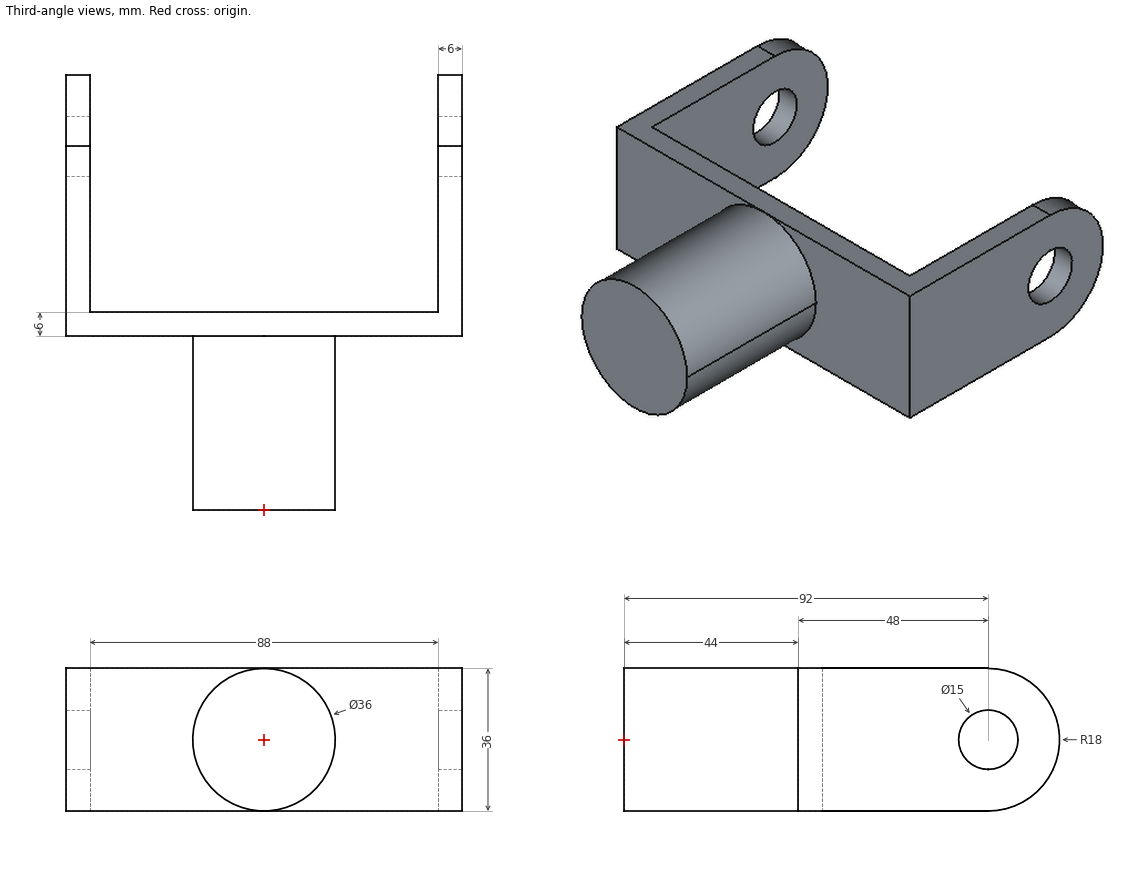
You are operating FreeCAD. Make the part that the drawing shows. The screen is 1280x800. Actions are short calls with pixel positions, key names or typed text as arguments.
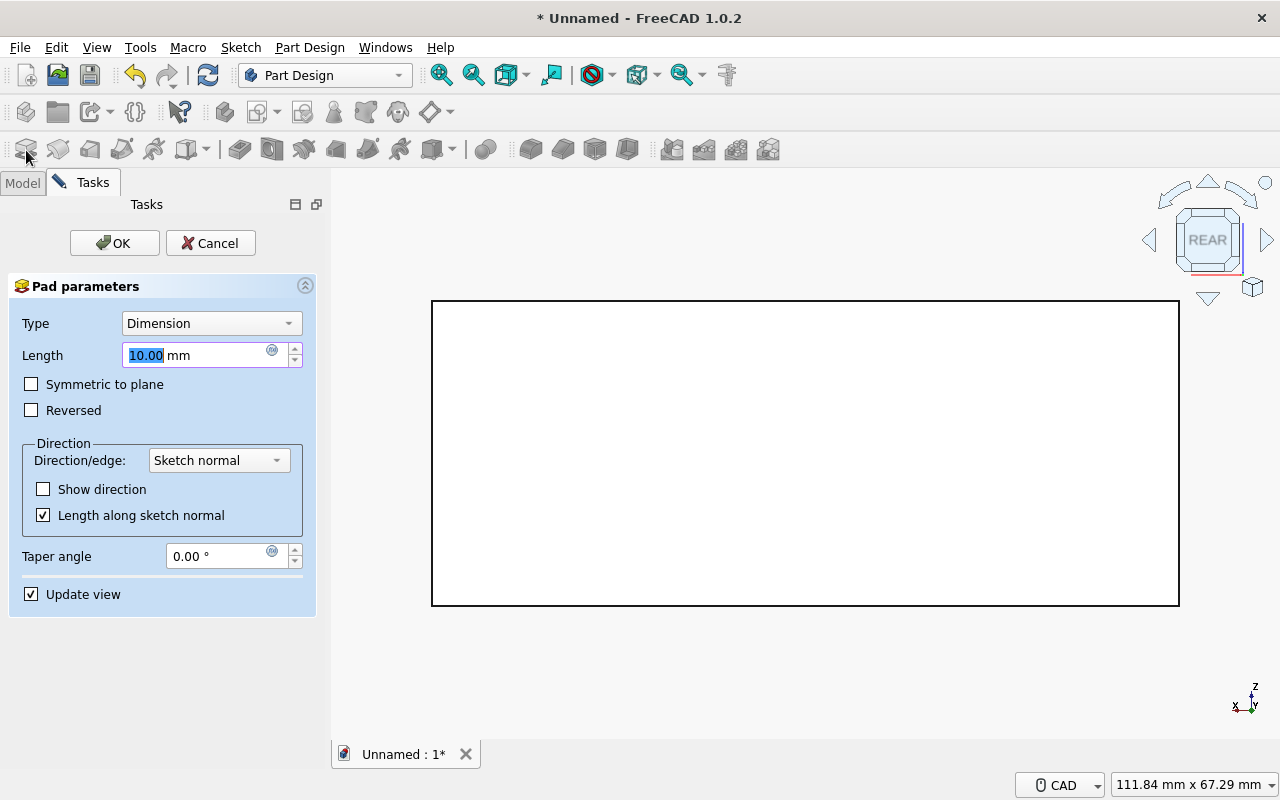
text(6)
key(Tab)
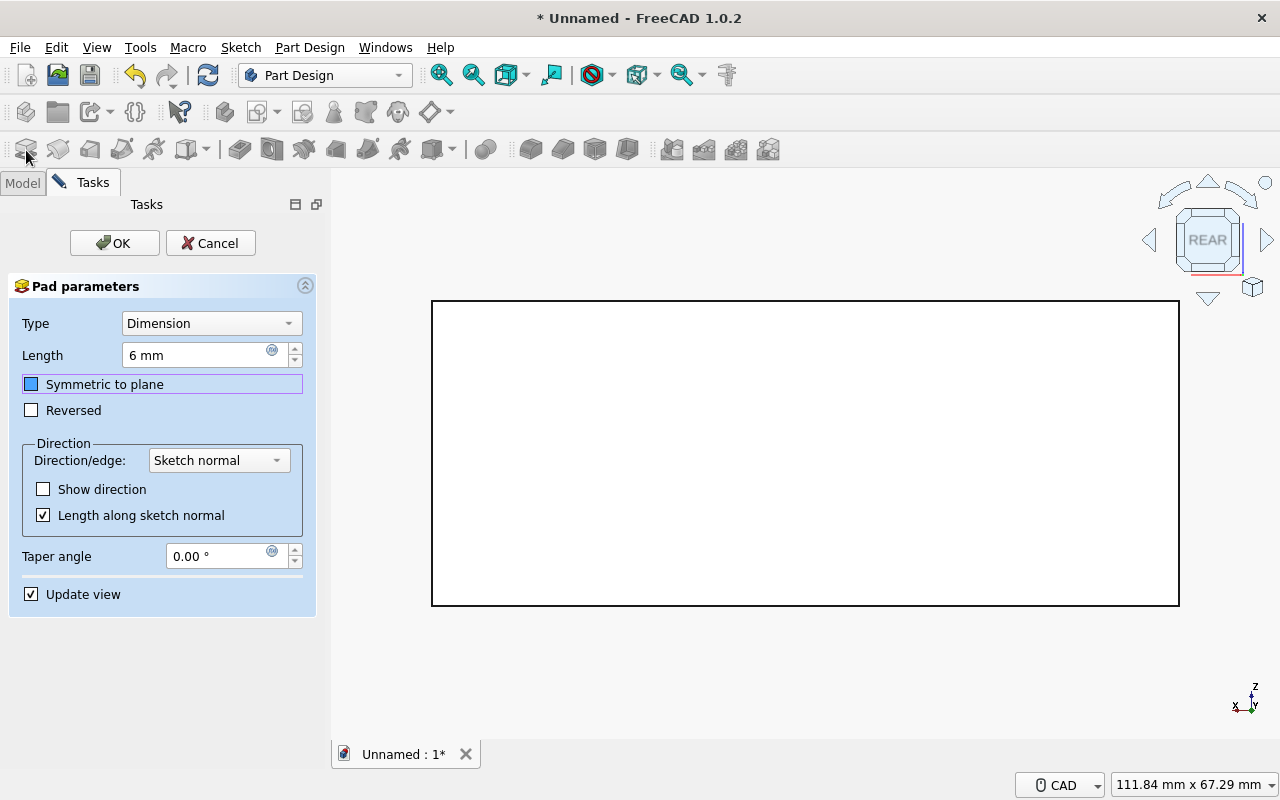
click(115, 243)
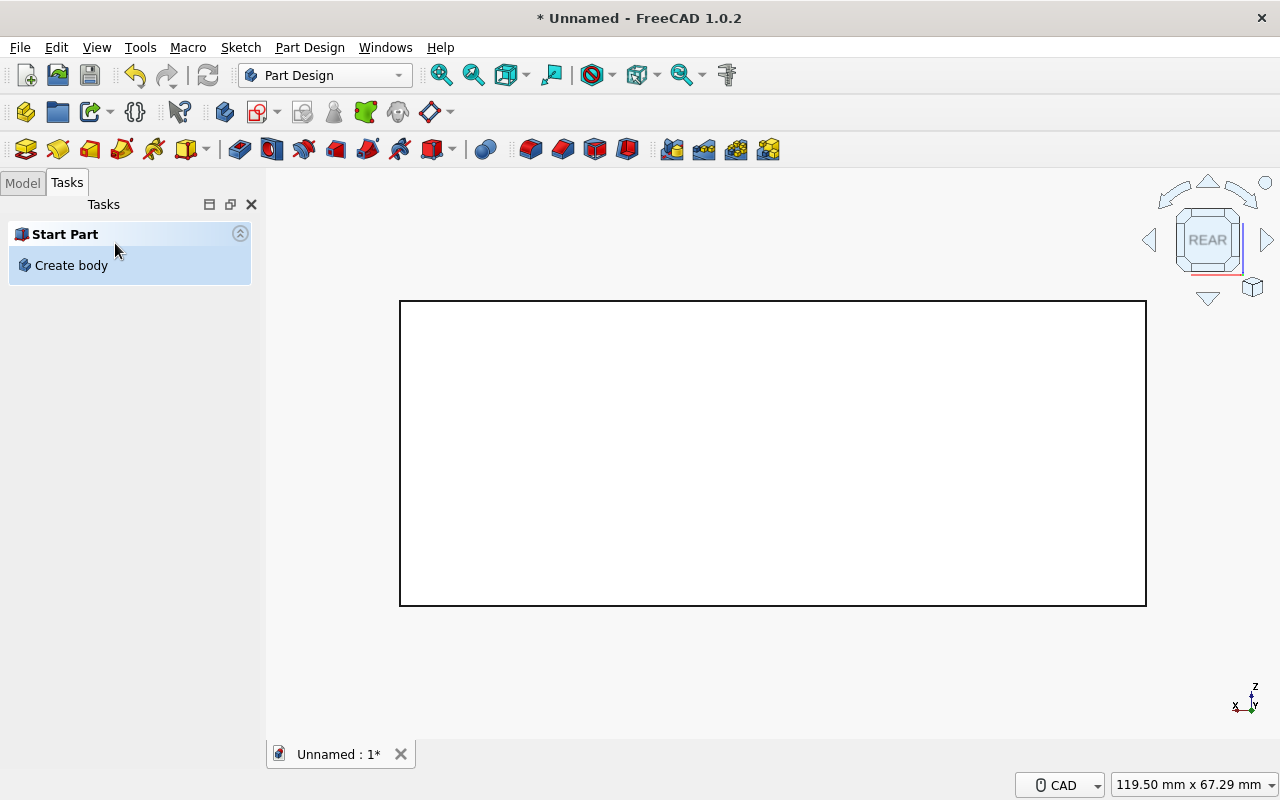
key(0)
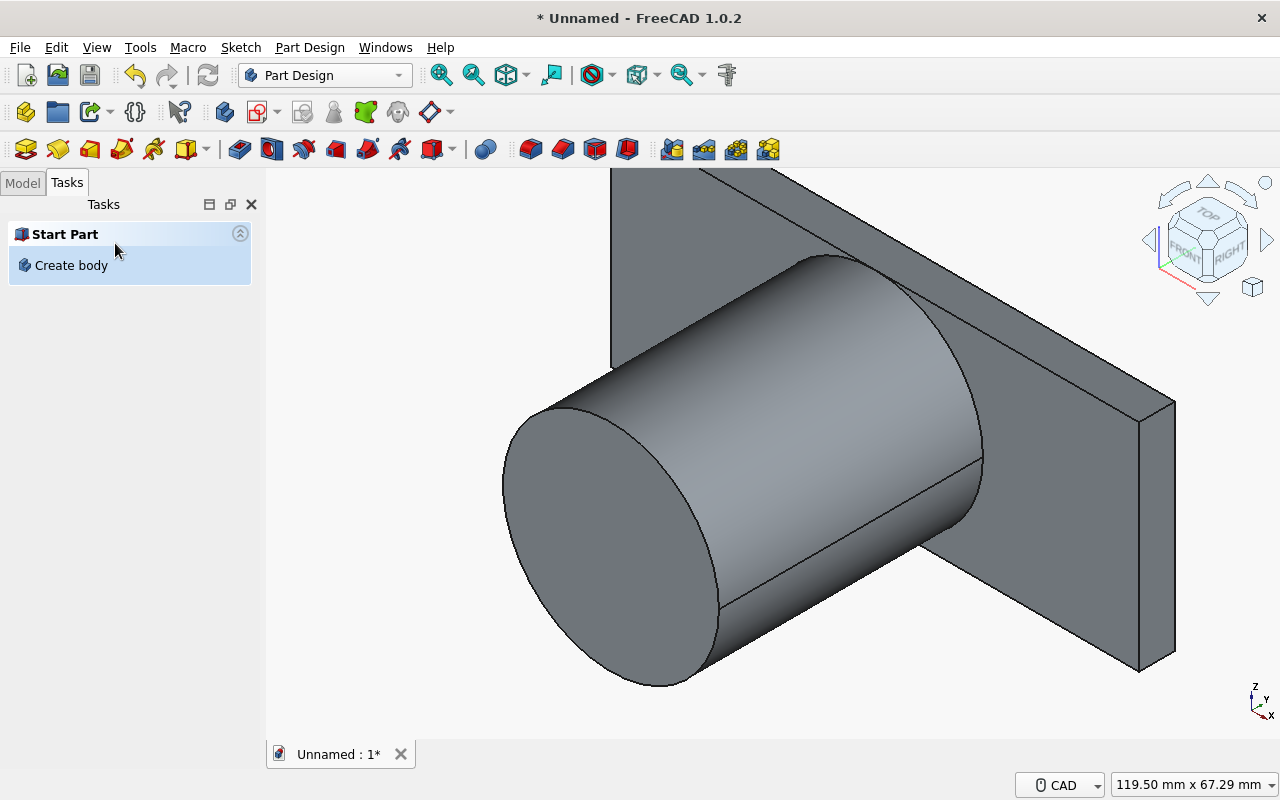
key(v)
key(f)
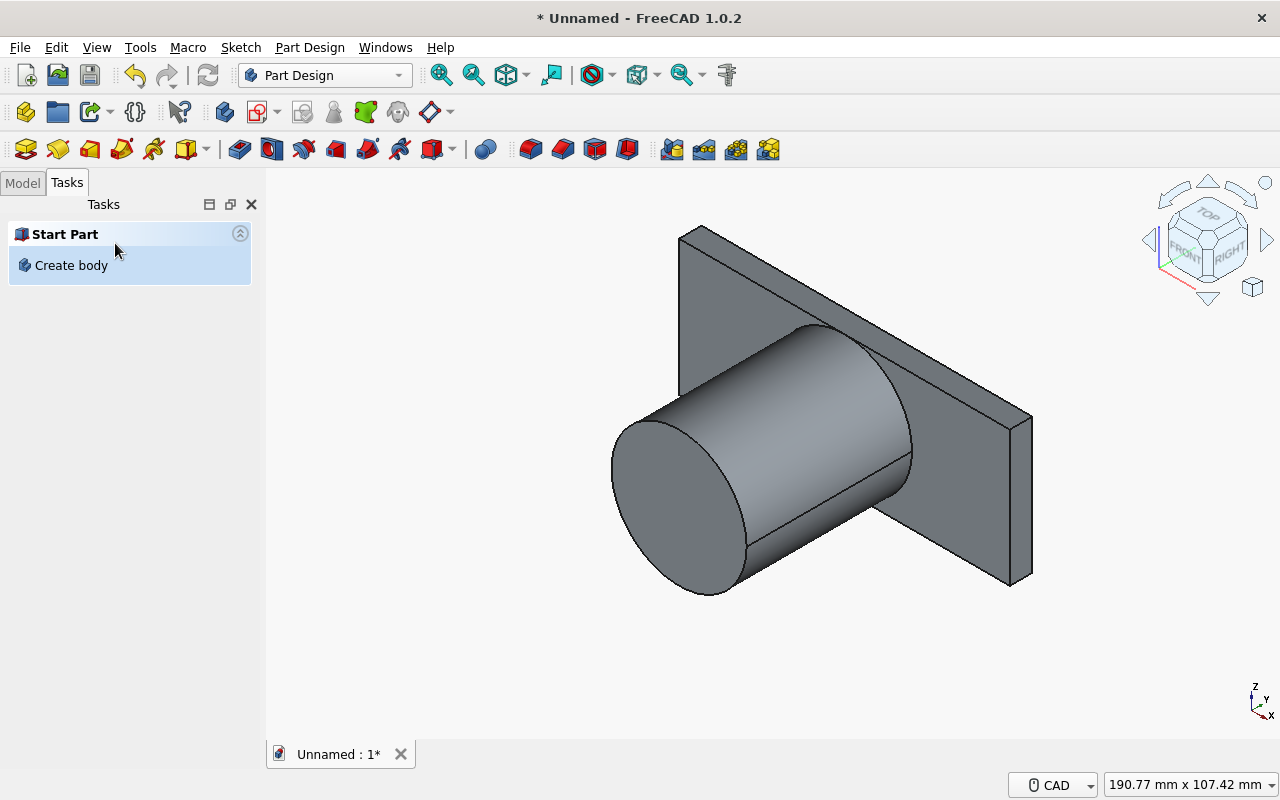
click(1021, 500)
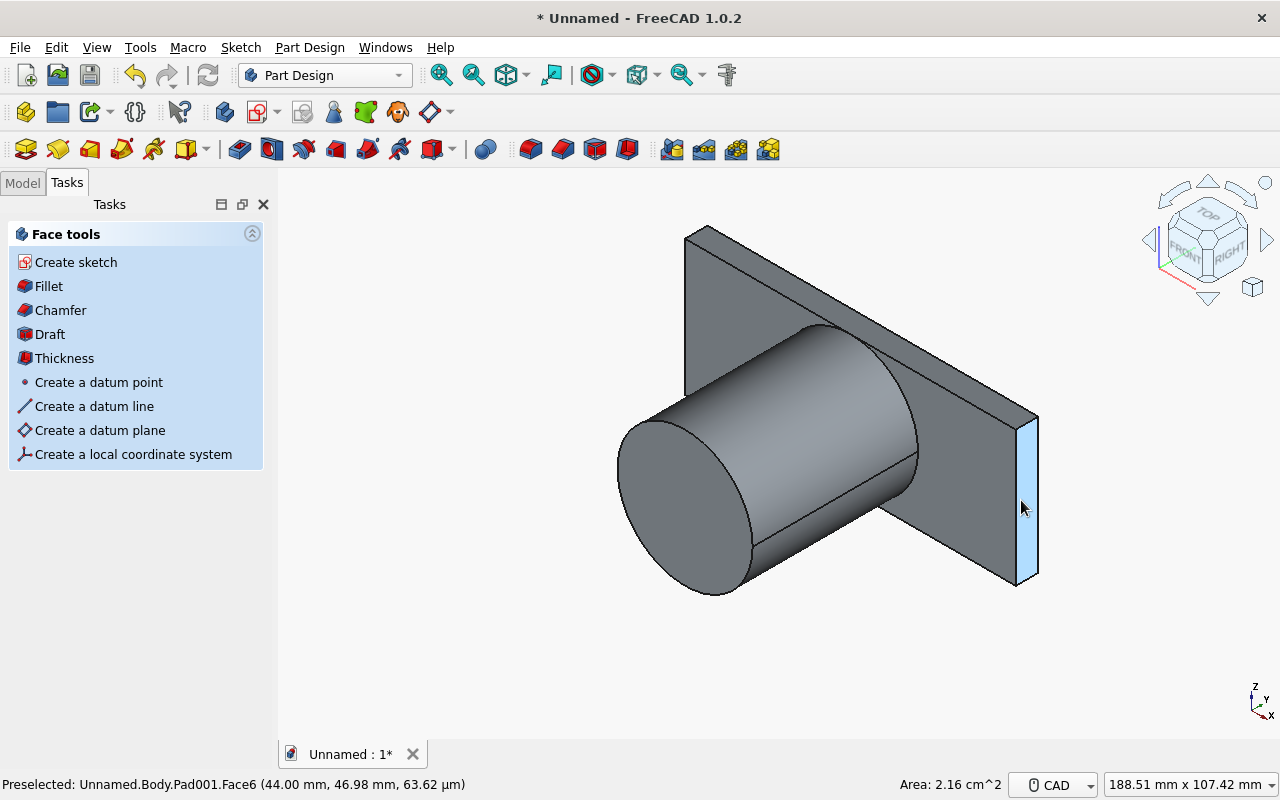
click(258, 112)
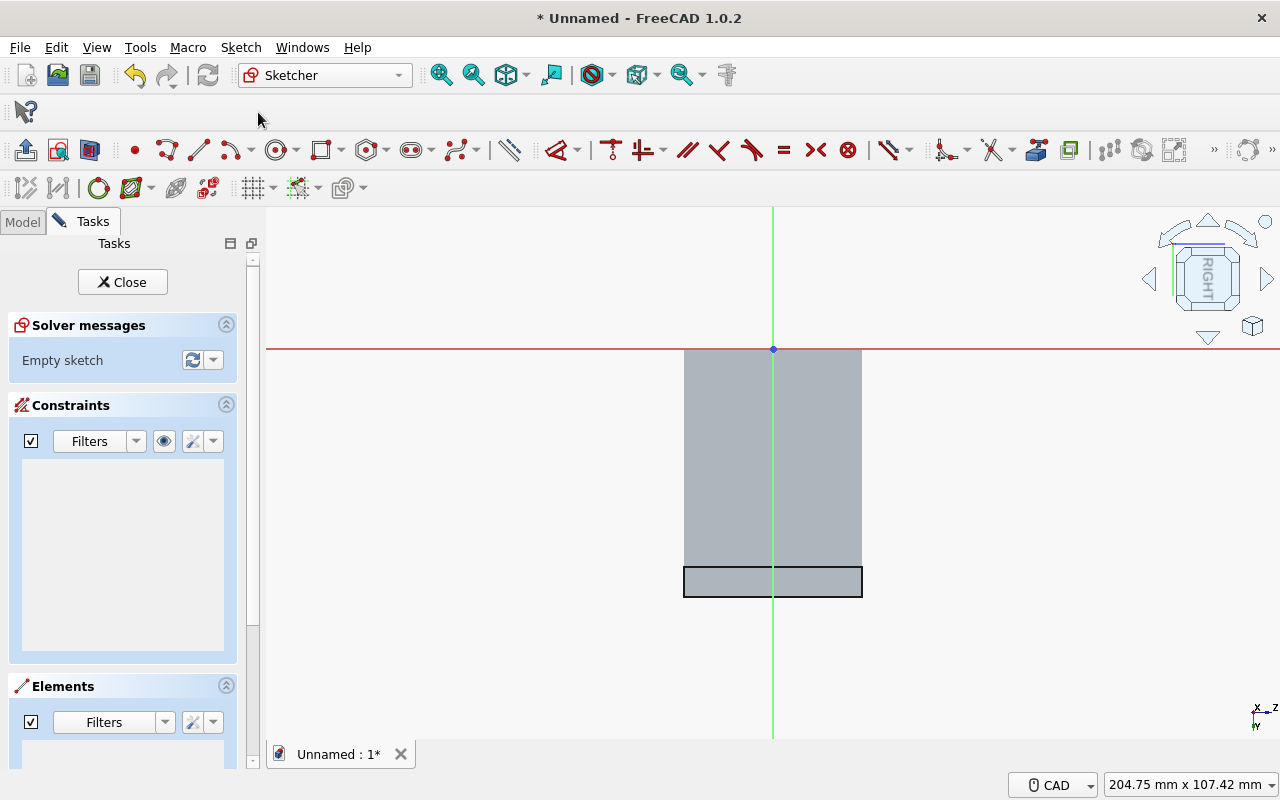
scroll(565, 235, down, 2)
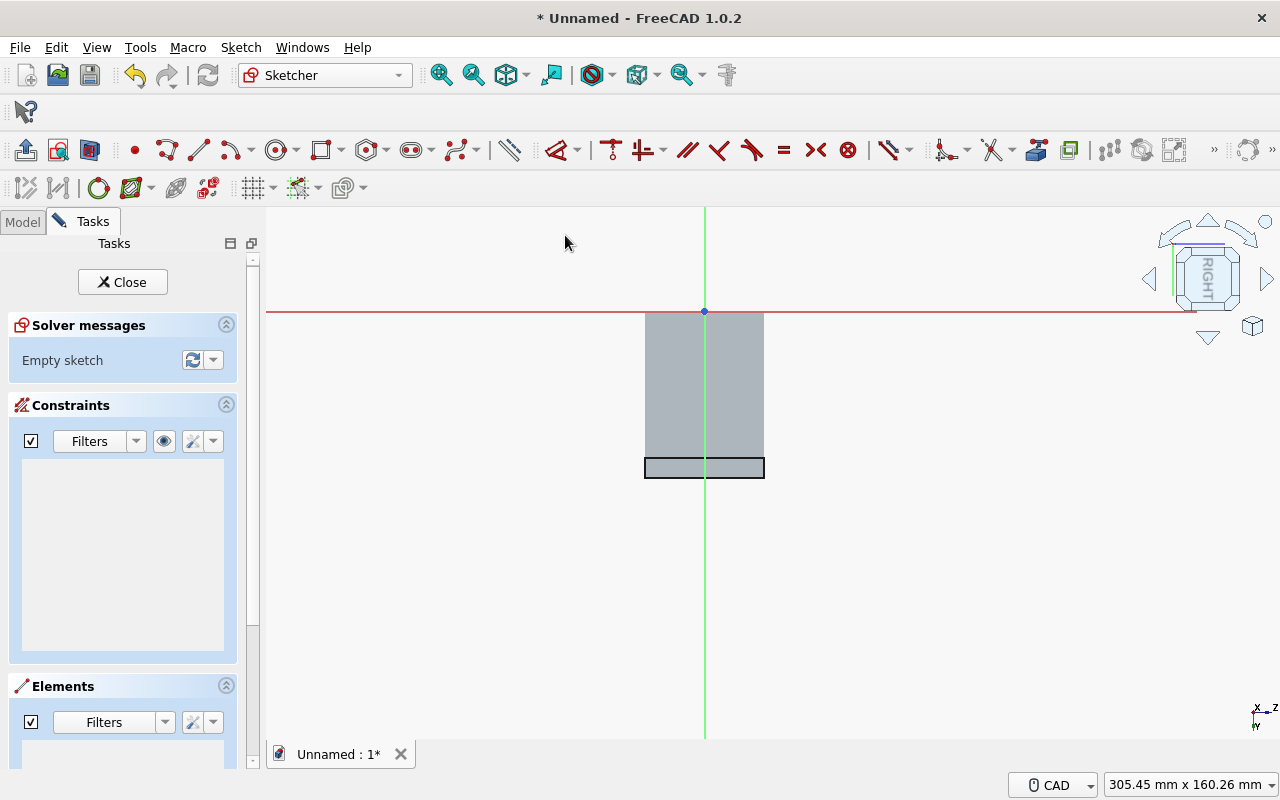
click(168, 150)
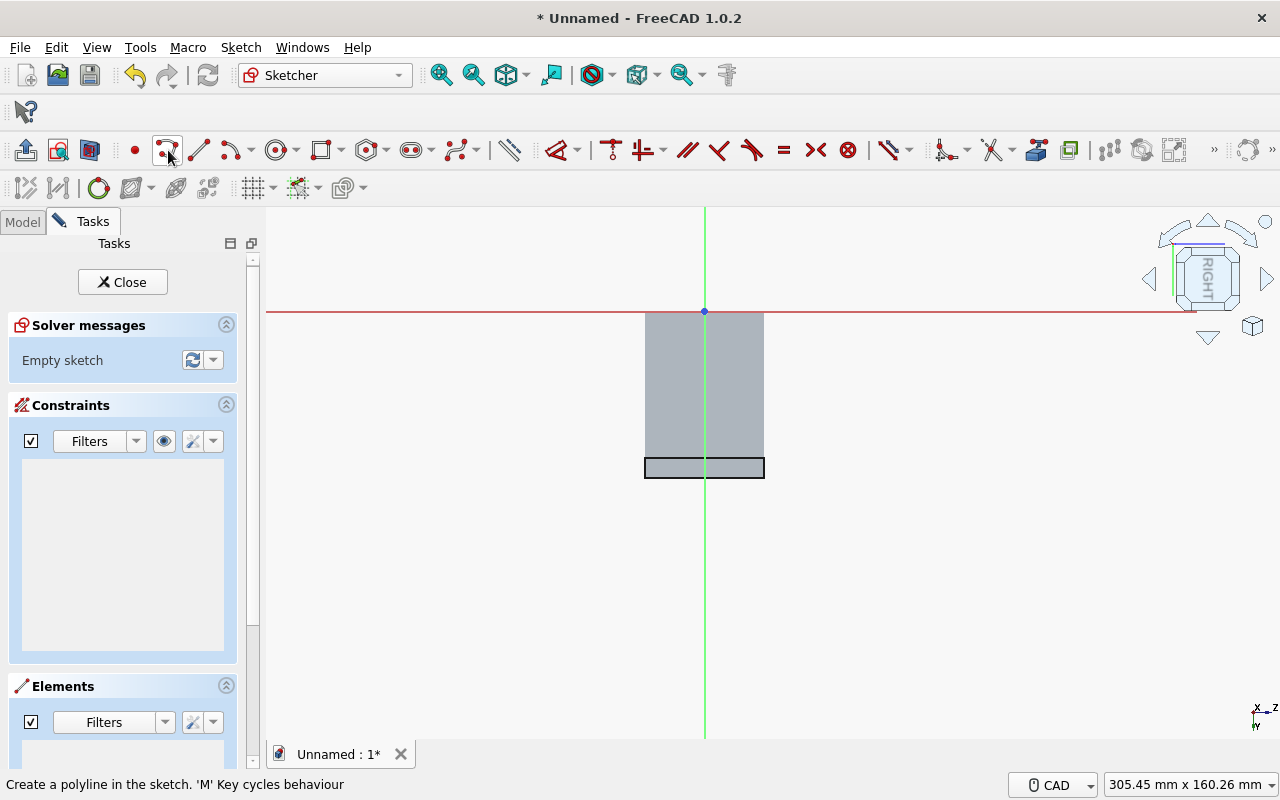
click(764, 617)
click(764, 458)
click(645, 458)
click(645, 617)
right_click(645, 617)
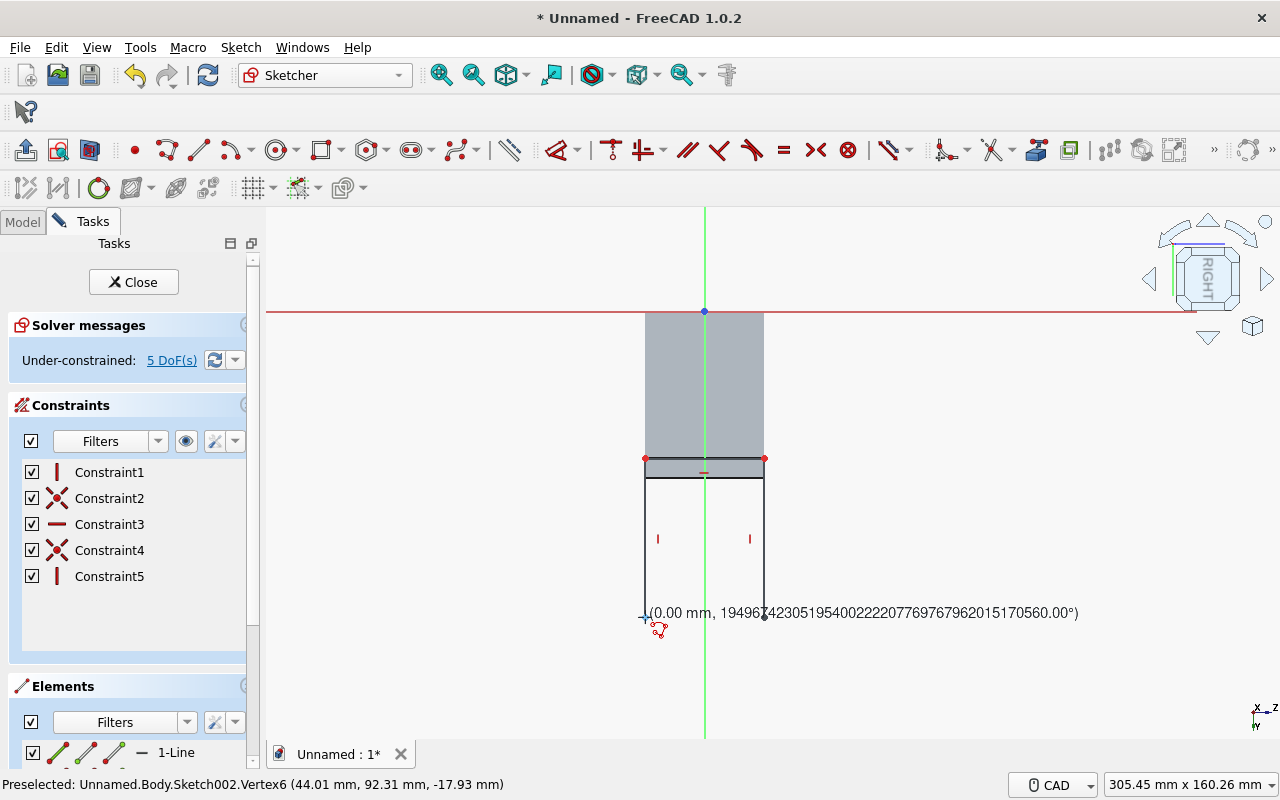
key(g)
key(3)
key(a)